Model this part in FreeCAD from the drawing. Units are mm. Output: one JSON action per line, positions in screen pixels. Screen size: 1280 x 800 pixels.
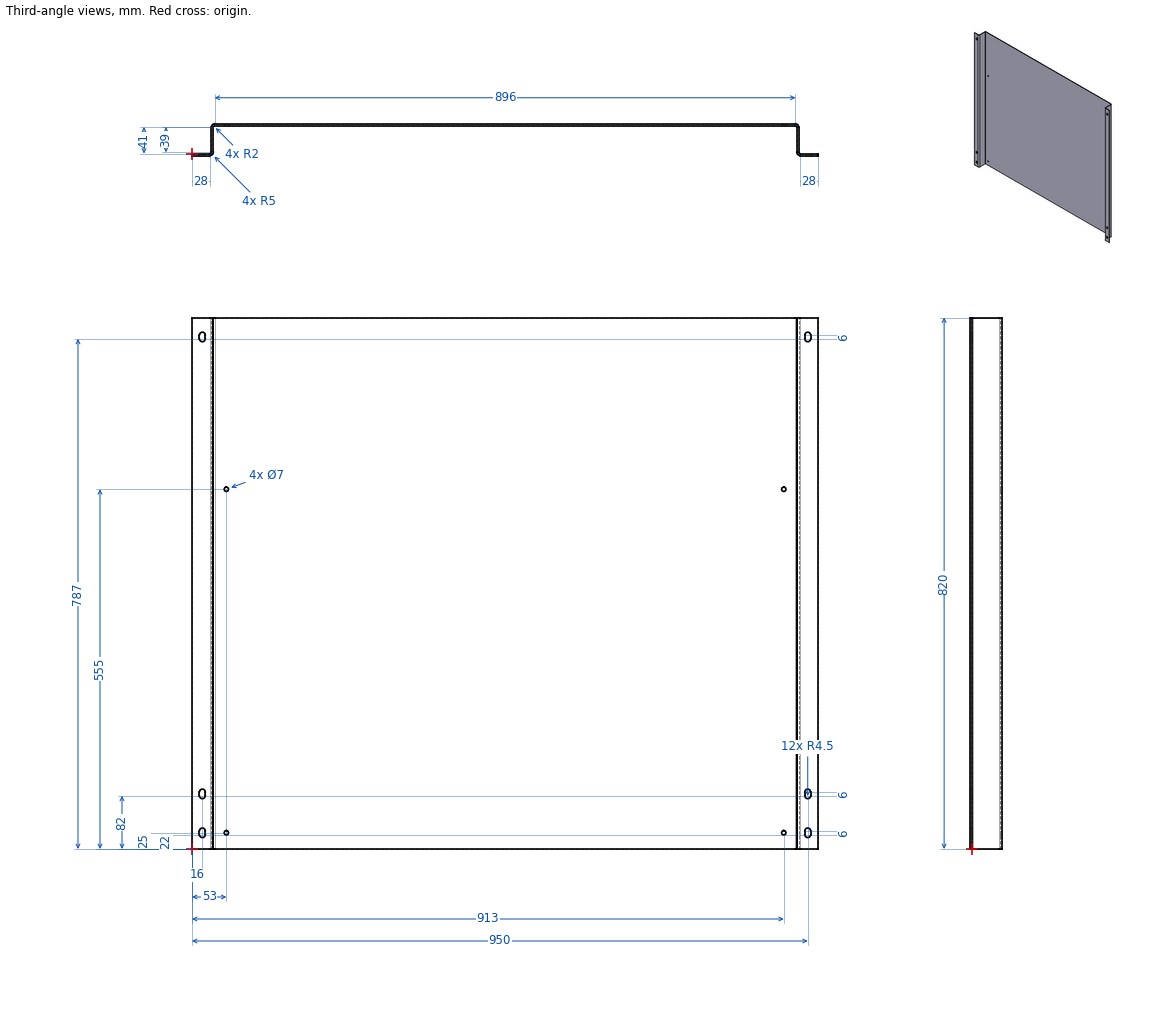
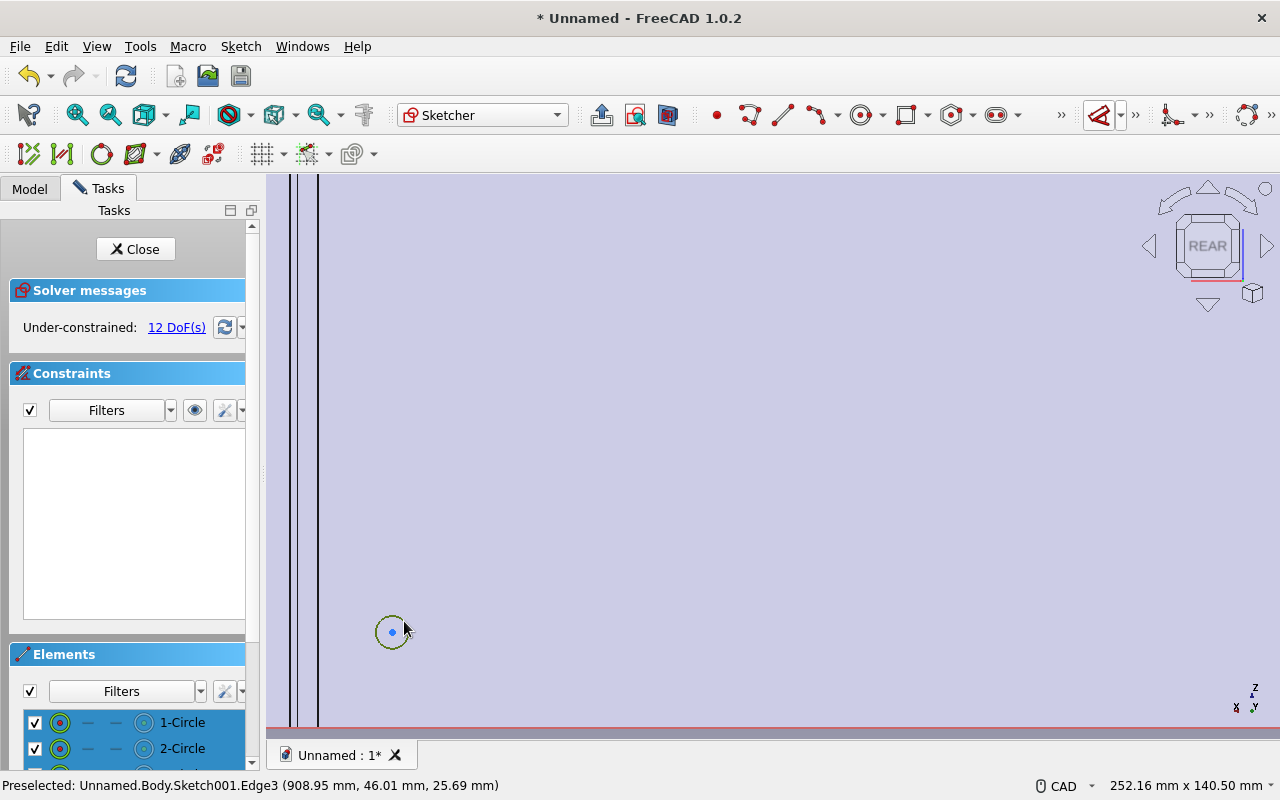
{"action": "scroll", "coordinate": [405, 625], "scroll_direction": "down", "scroll_amount": 9}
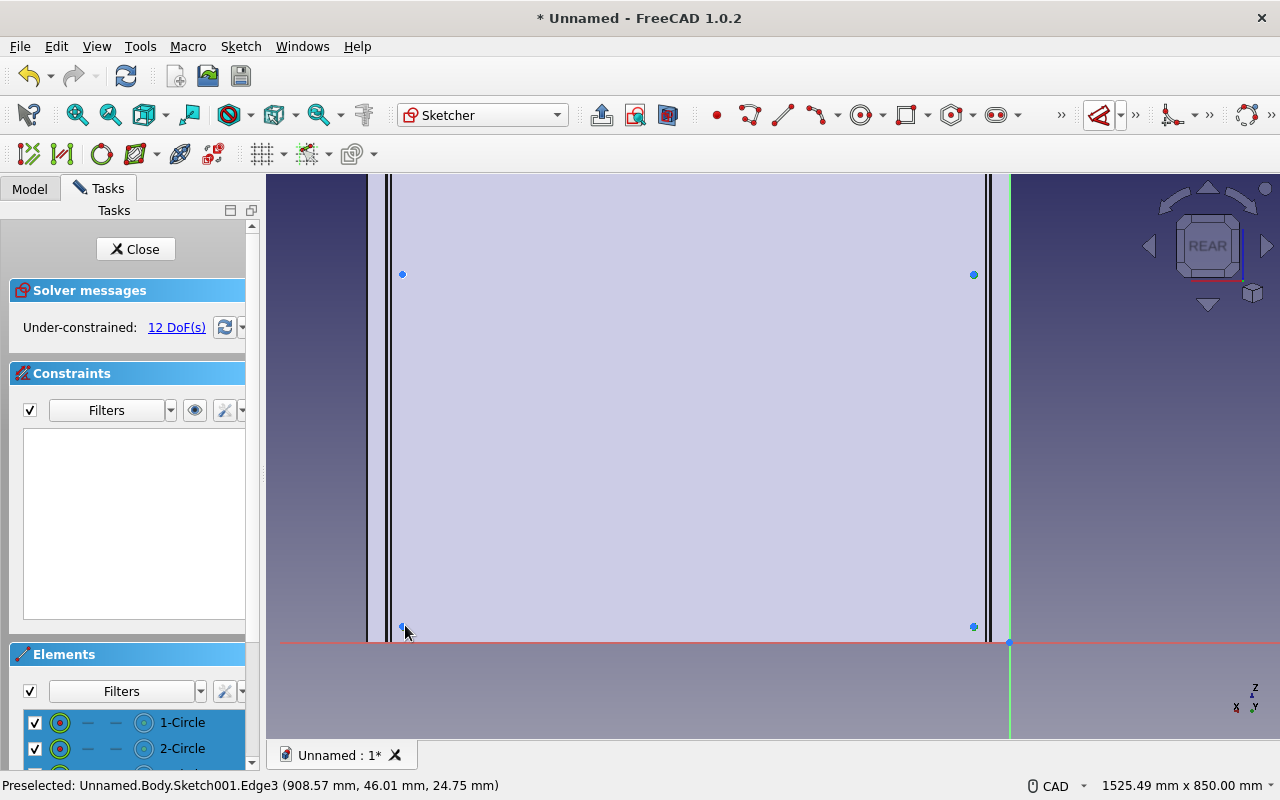
{"action": "scroll", "coordinate": [405, 273], "scroll_direction": "up", "scroll_amount": 8}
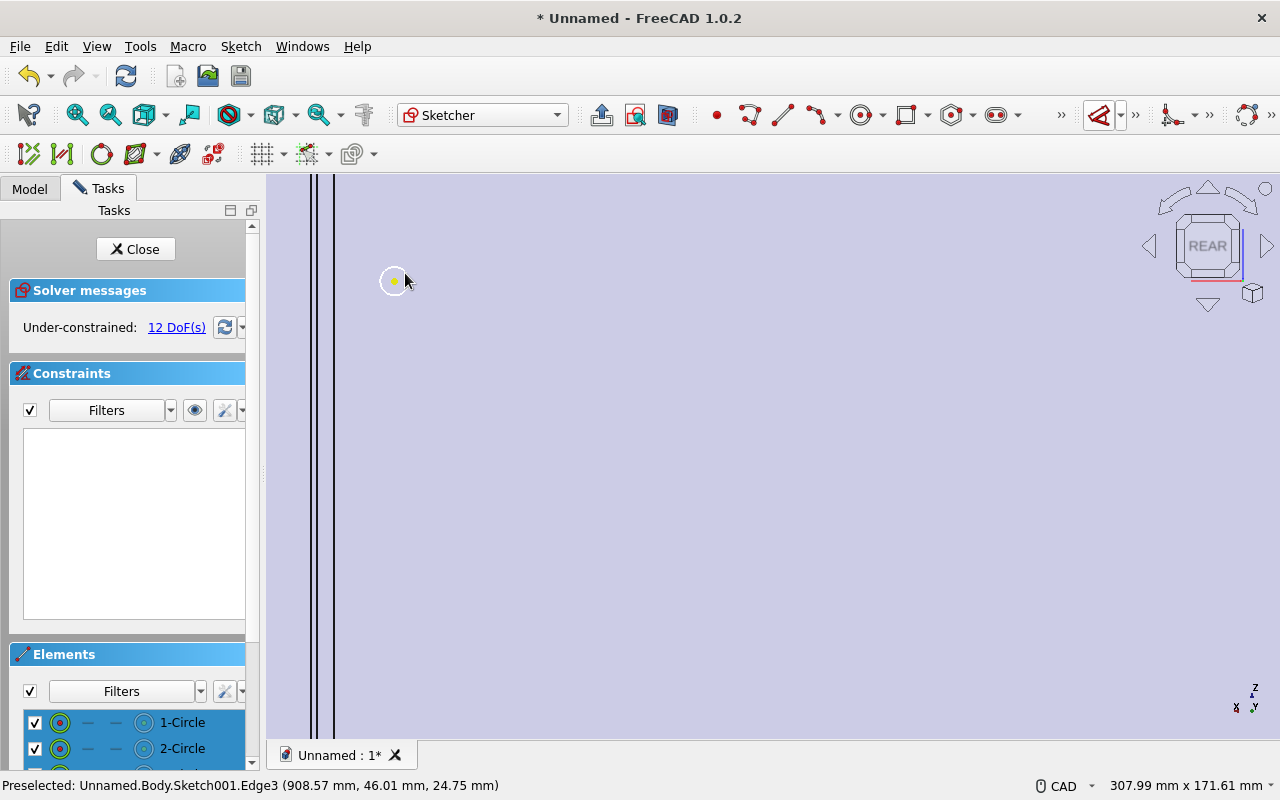
{"action": "left_click", "coordinate": [405, 271]}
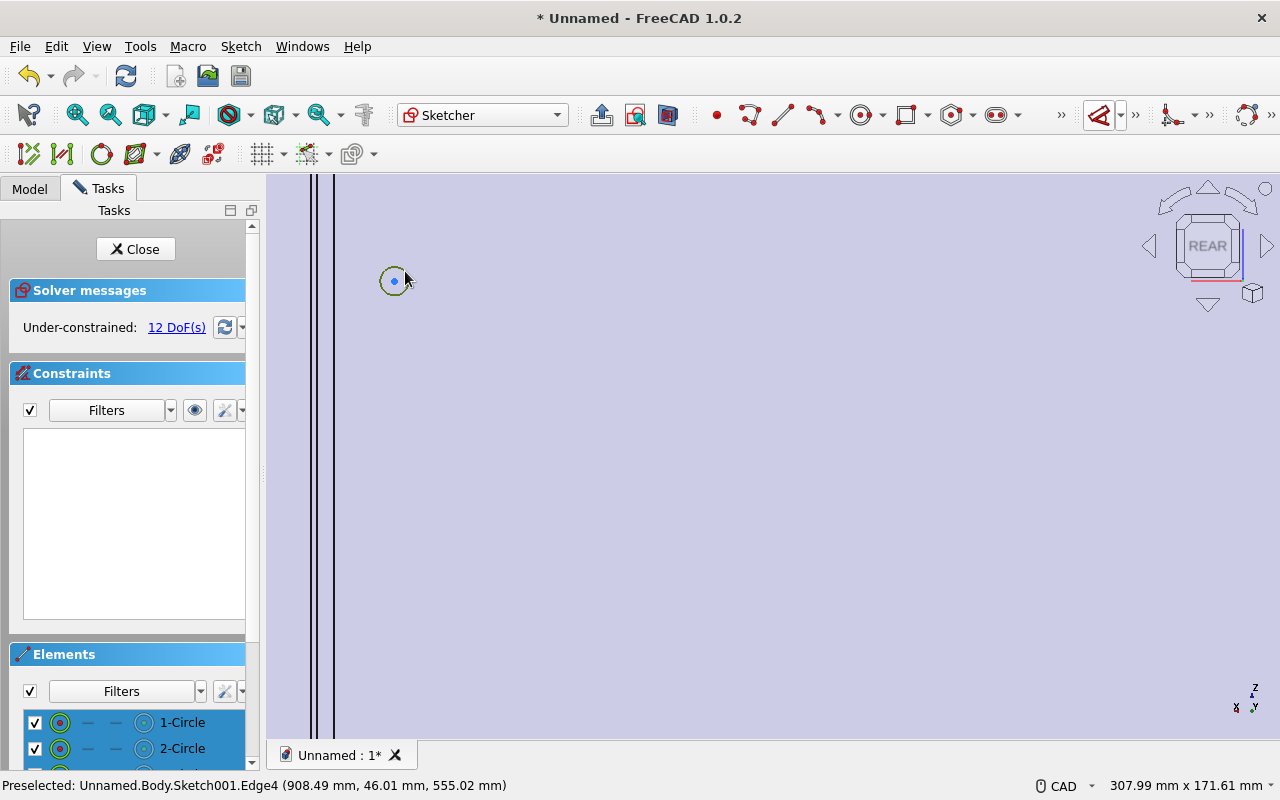
{"action": "key", "text": "e"}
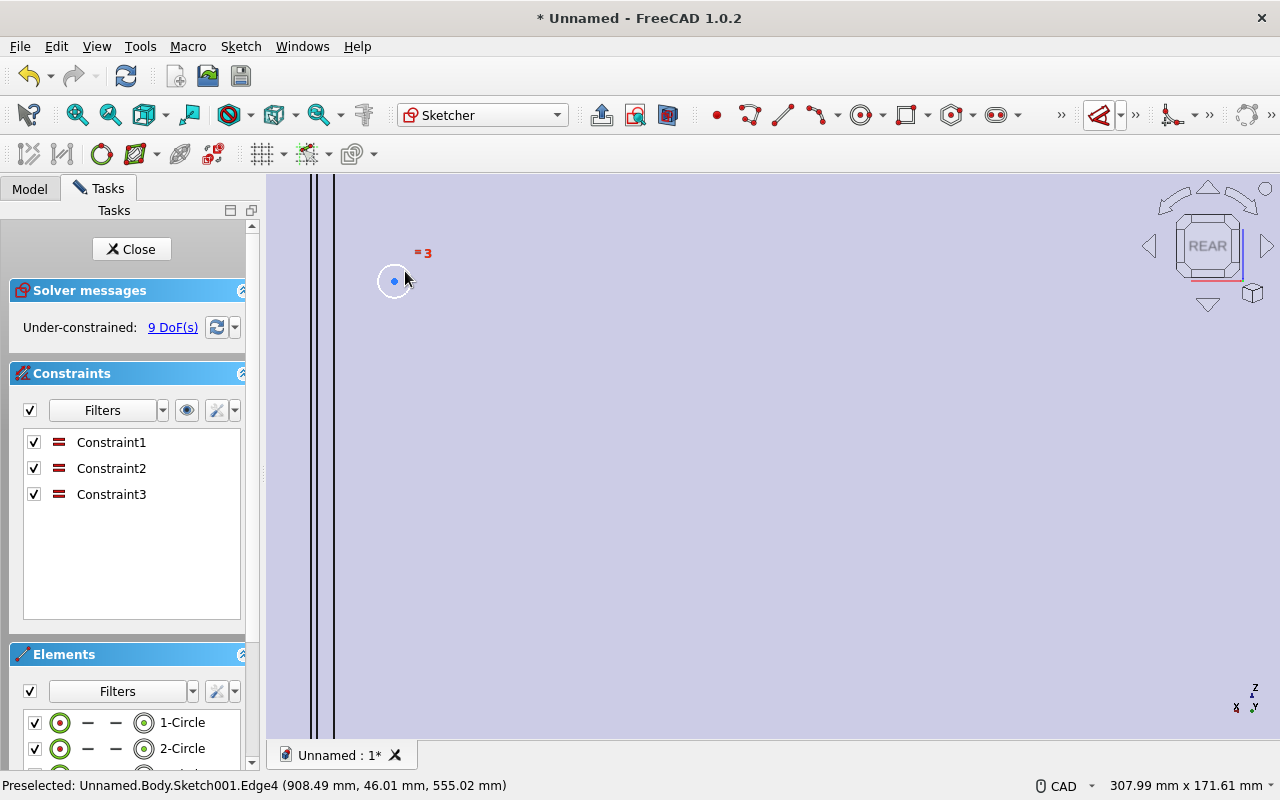
{"action": "key", "text": "d"}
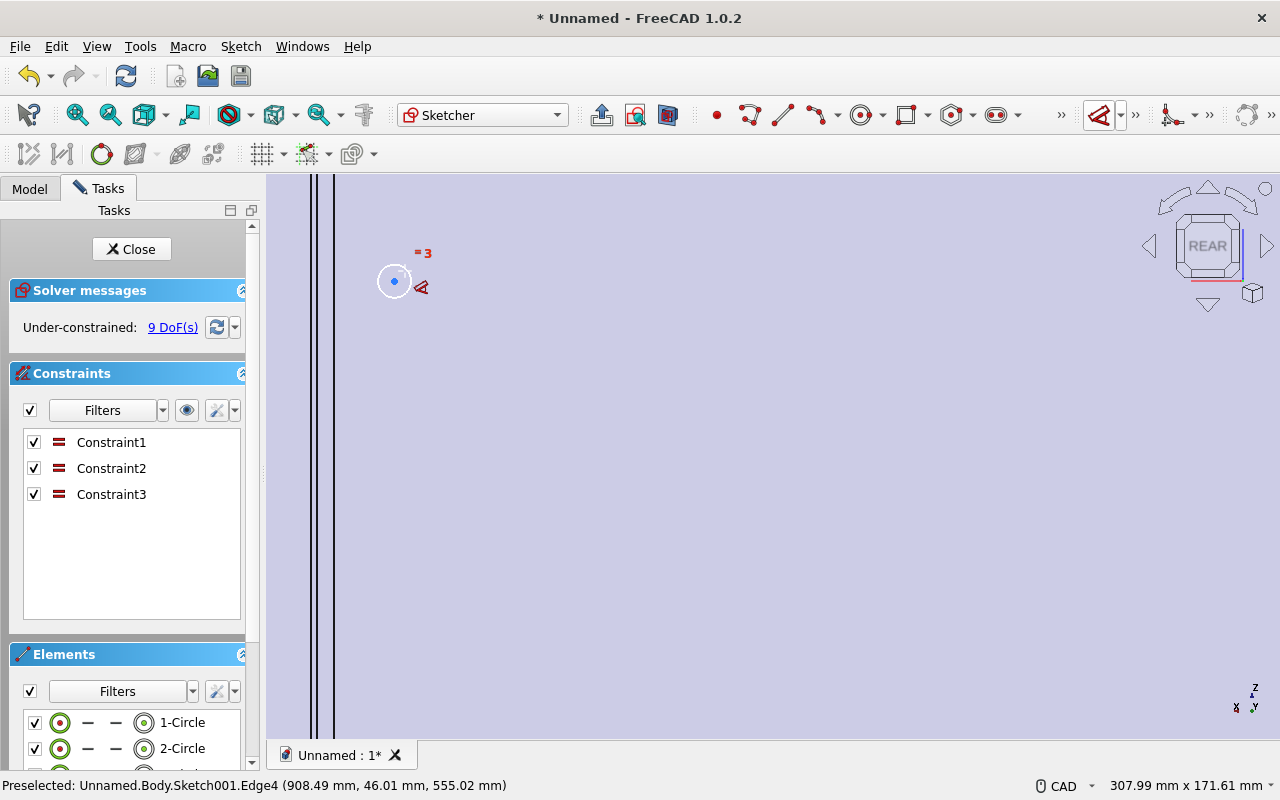
{"action": "scroll", "coordinate": [405, 272], "scroll_direction": "down", "scroll_amount": 8}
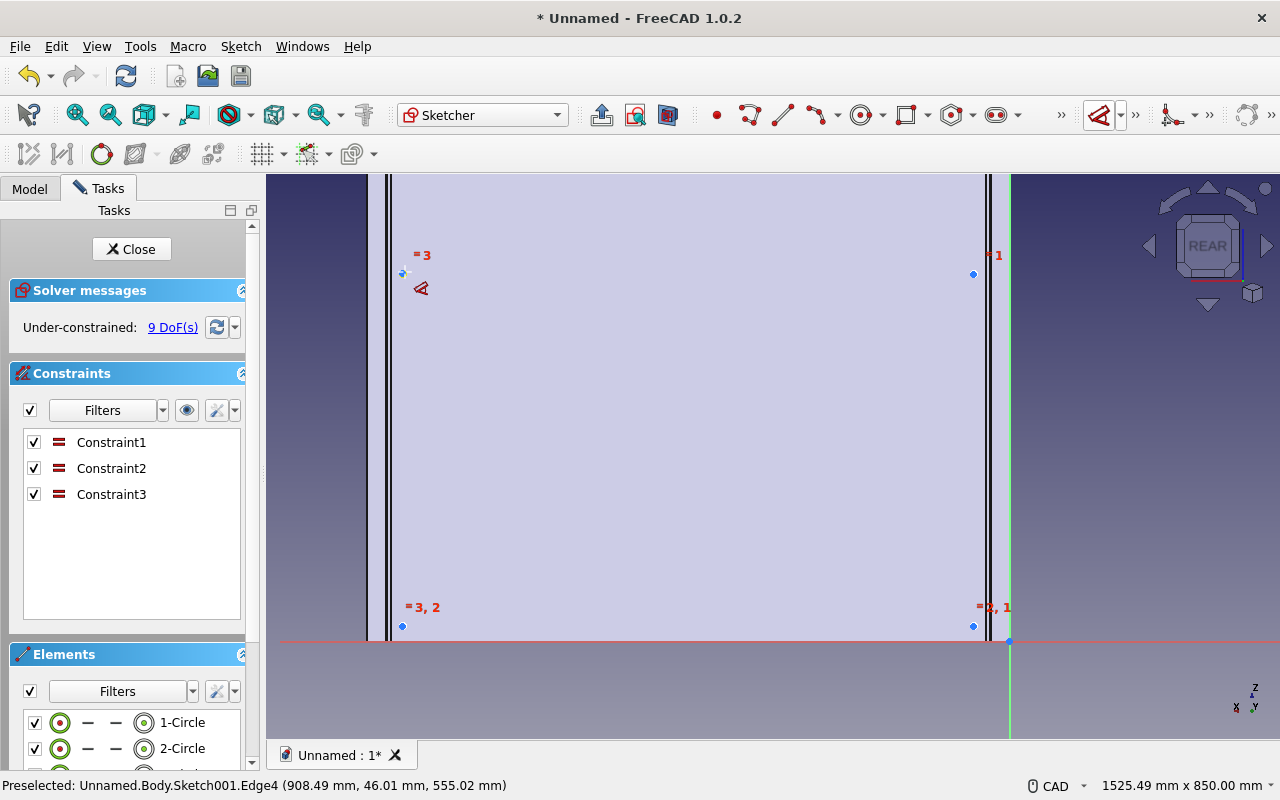
{"action": "scroll", "coordinate": [976, 272], "scroll_direction": "up", "scroll_amount": 11}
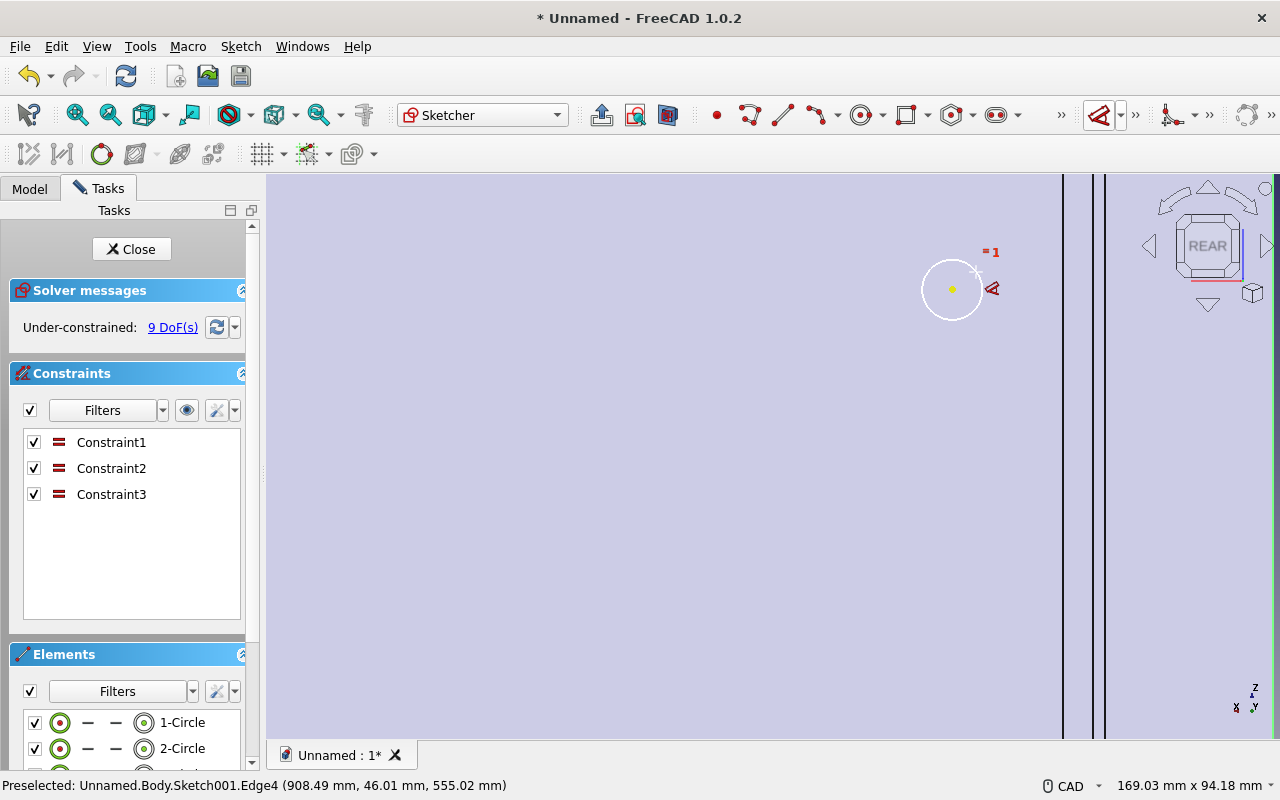
{"action": "left_click", "coordinate": [974, 269]}
{"action": "left_click", "coordinate": [997, 247]}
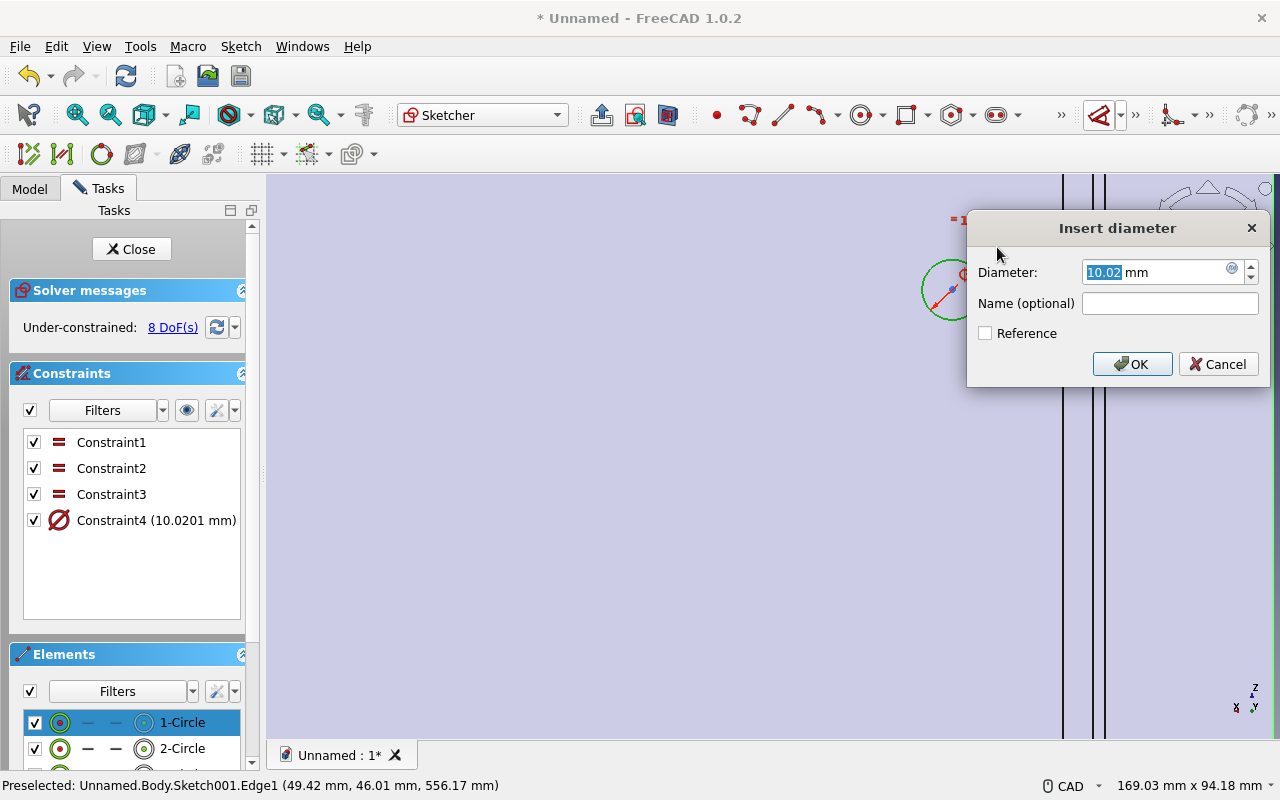
{"action": "type", "text": "7"}
{"action": "key", "text": "Return"}